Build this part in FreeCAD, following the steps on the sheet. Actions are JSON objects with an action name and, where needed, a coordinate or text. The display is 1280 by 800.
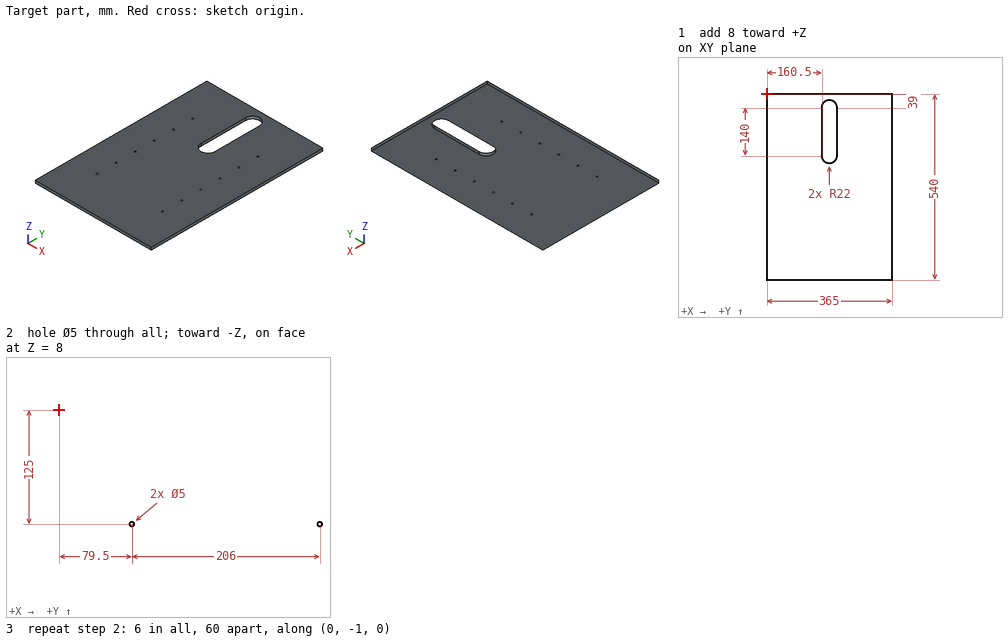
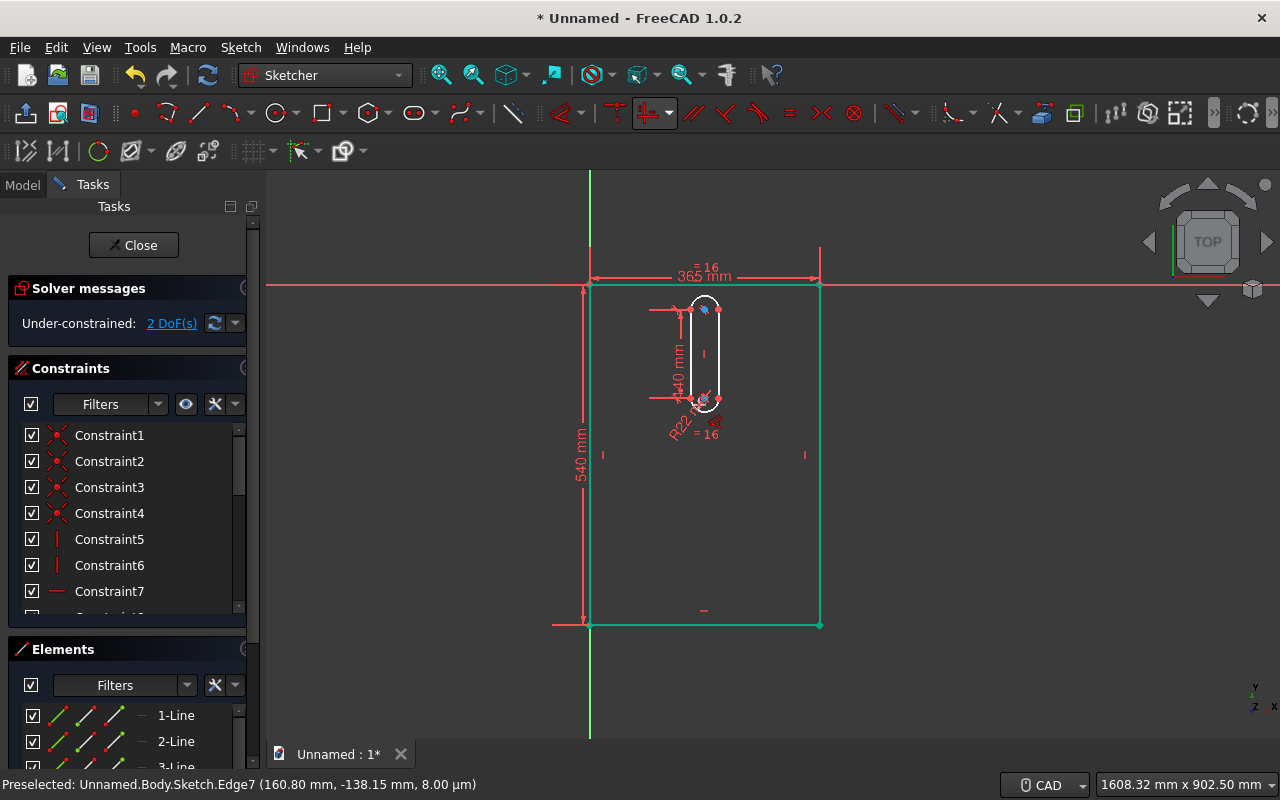
{"action": "scroll", "coordinate": [719, 310], "scroll_direction": "up", "scroll_amount": 3}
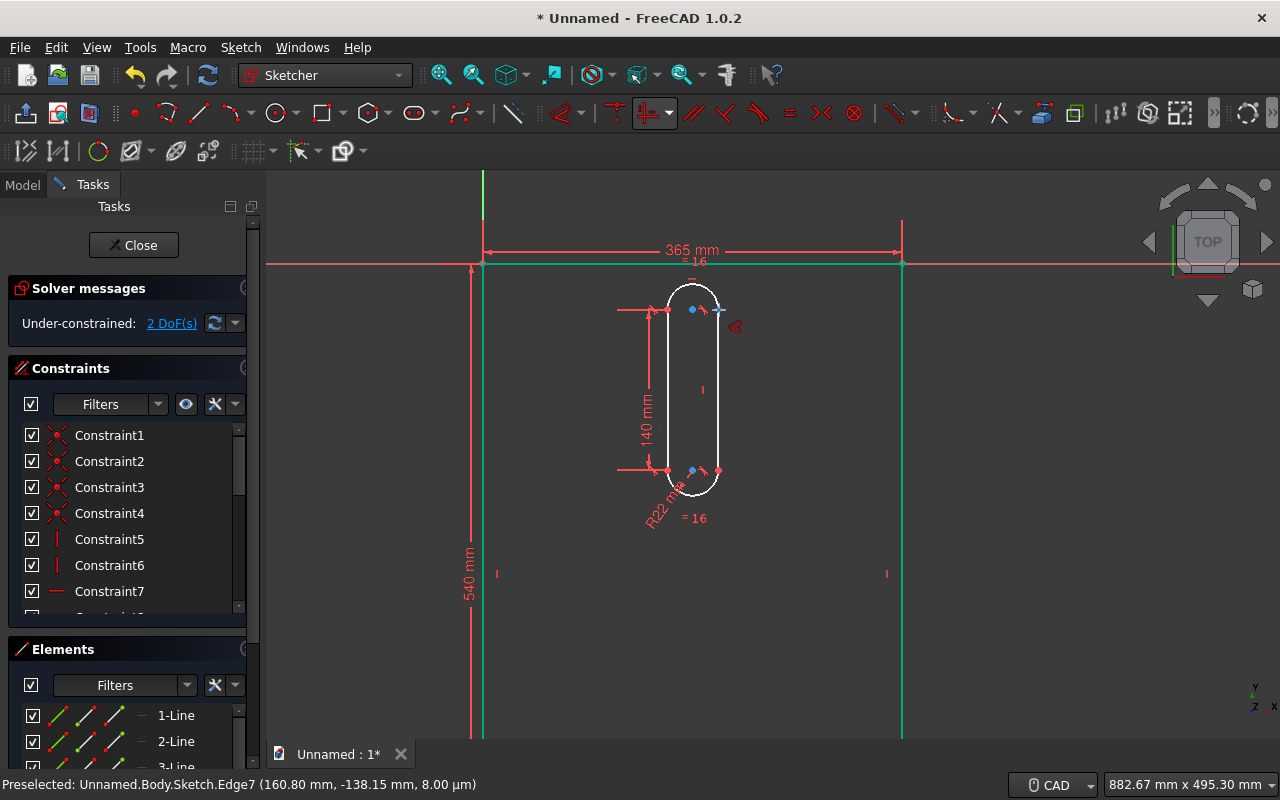
{"action": "left_click", "coordinate": [718, 310]}
{"action": "left_click", "coordinate": [449, 287]}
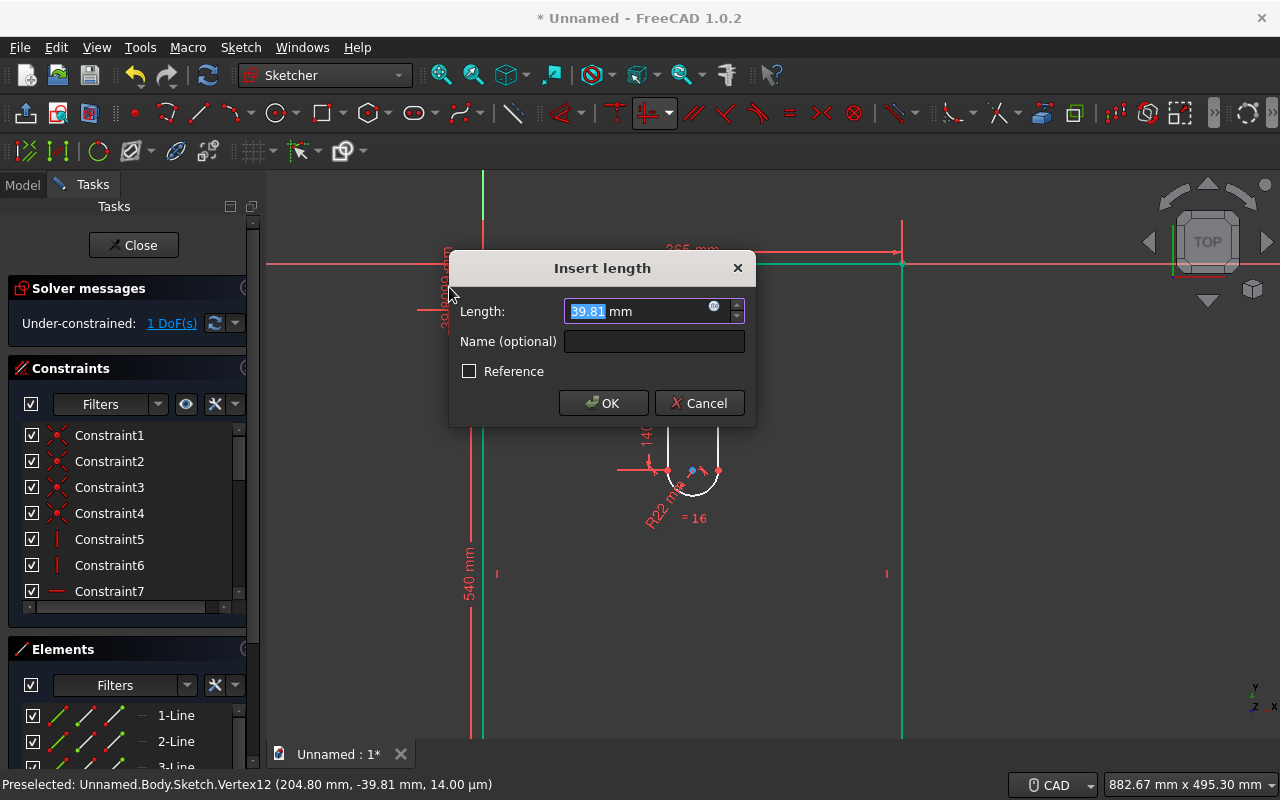
{"action": "type", "text": "39"}
{"action": "key", "text": "Return"}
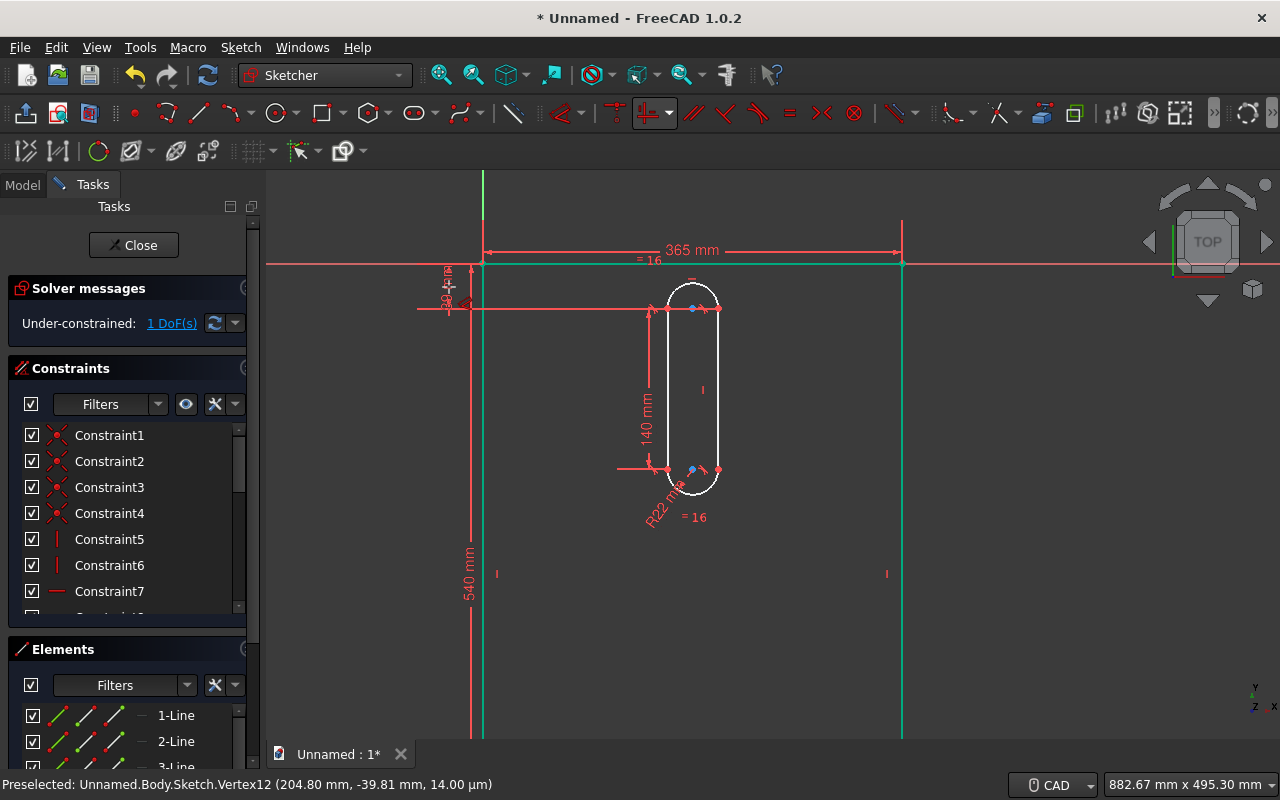
{"action": "left_click", "coordinate": [668, 469]}
{"action": "left_click", "coordinate": [575, 230]}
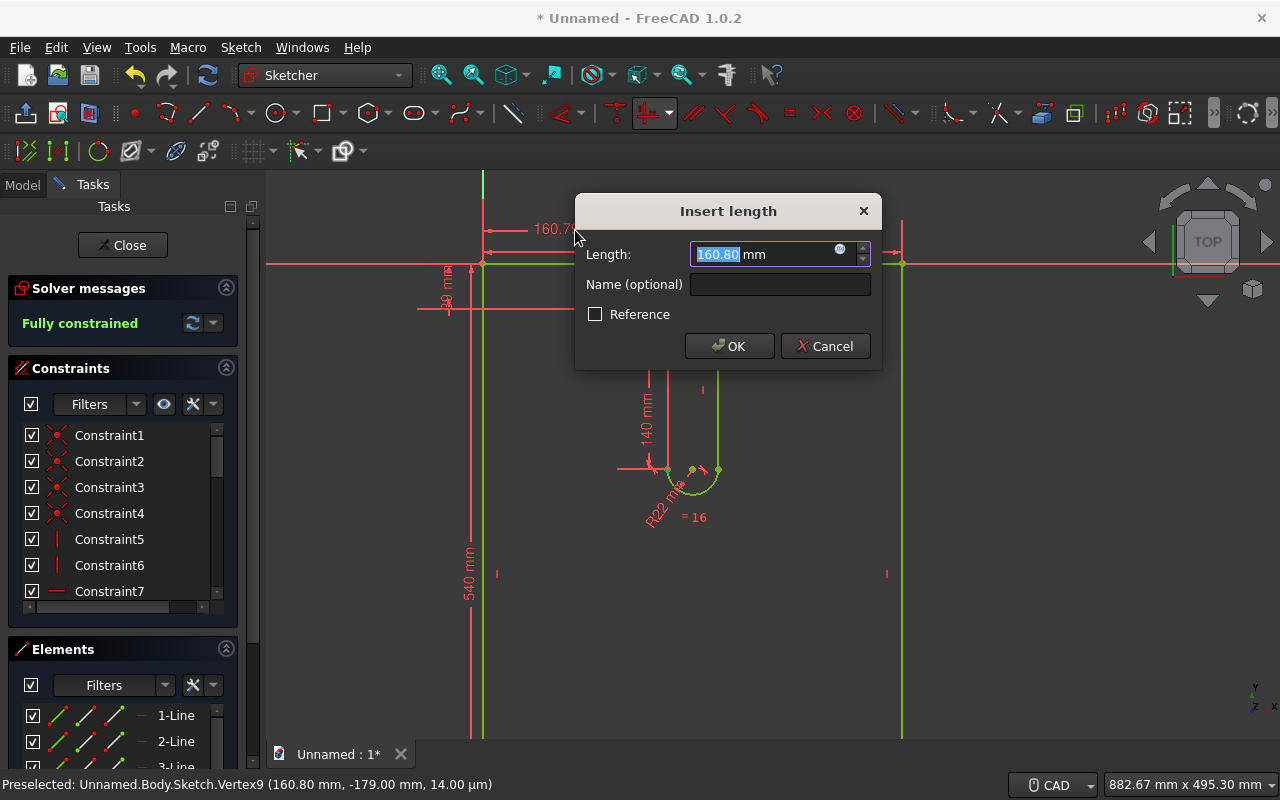
{"action": "type", "text": "160.5"}
{"action": "key", "text": "Return"}
{"action": "key", "text": "Escape"}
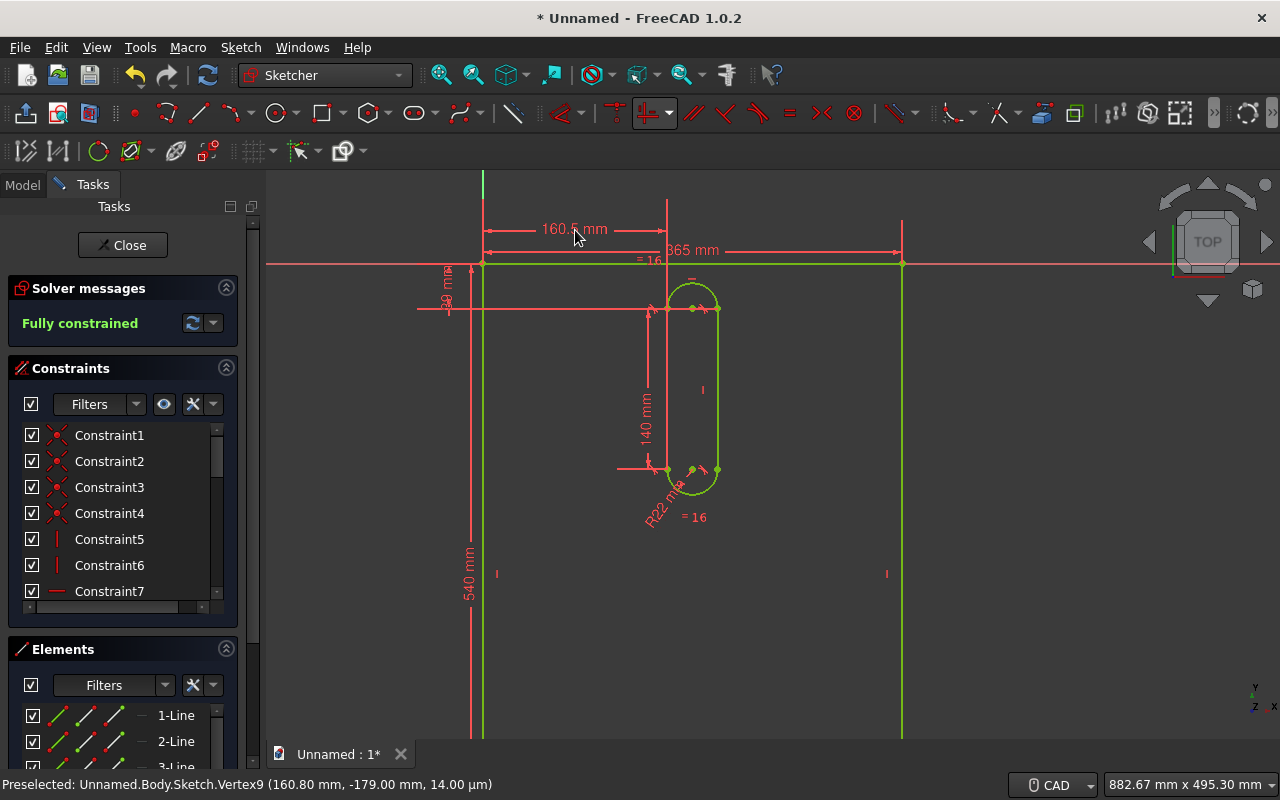
{"action": "left_click", "coordinate": [123, 245]}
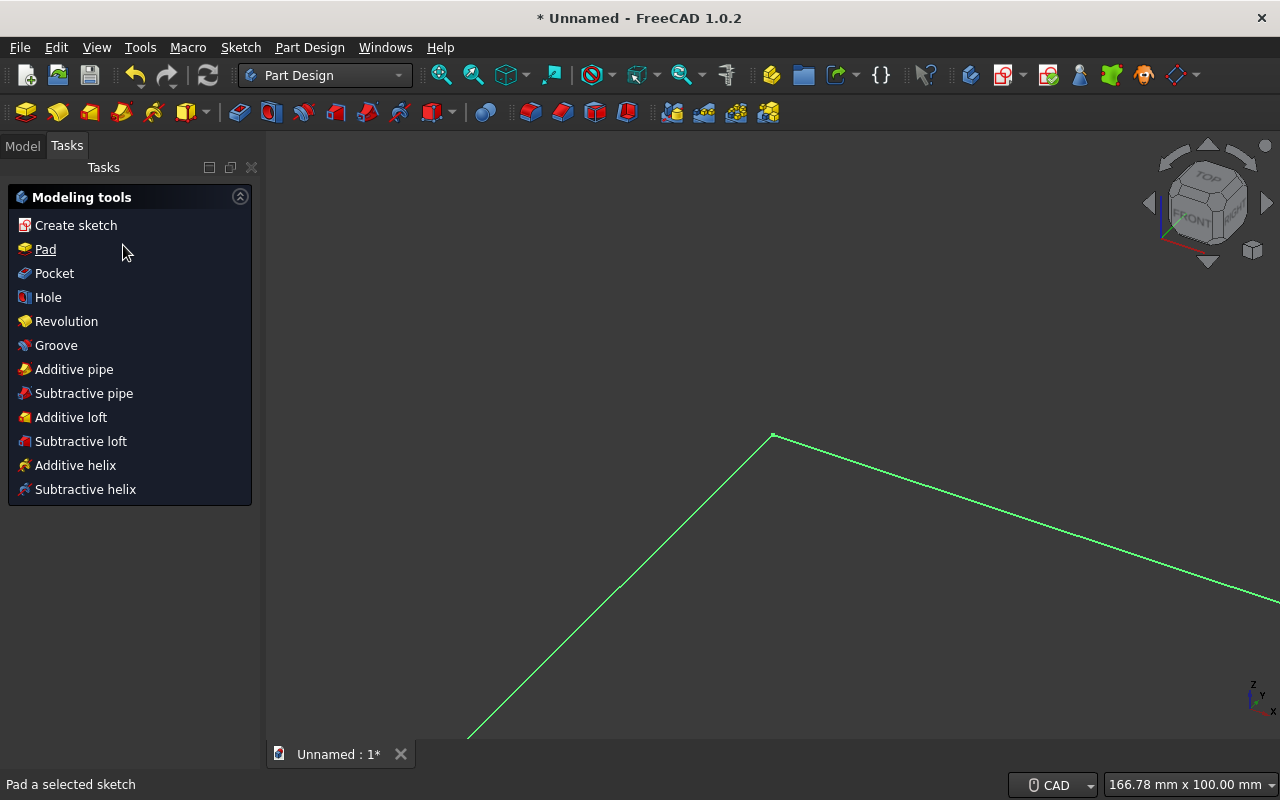
{"action": "left_click", "coordinate": [26, 112]}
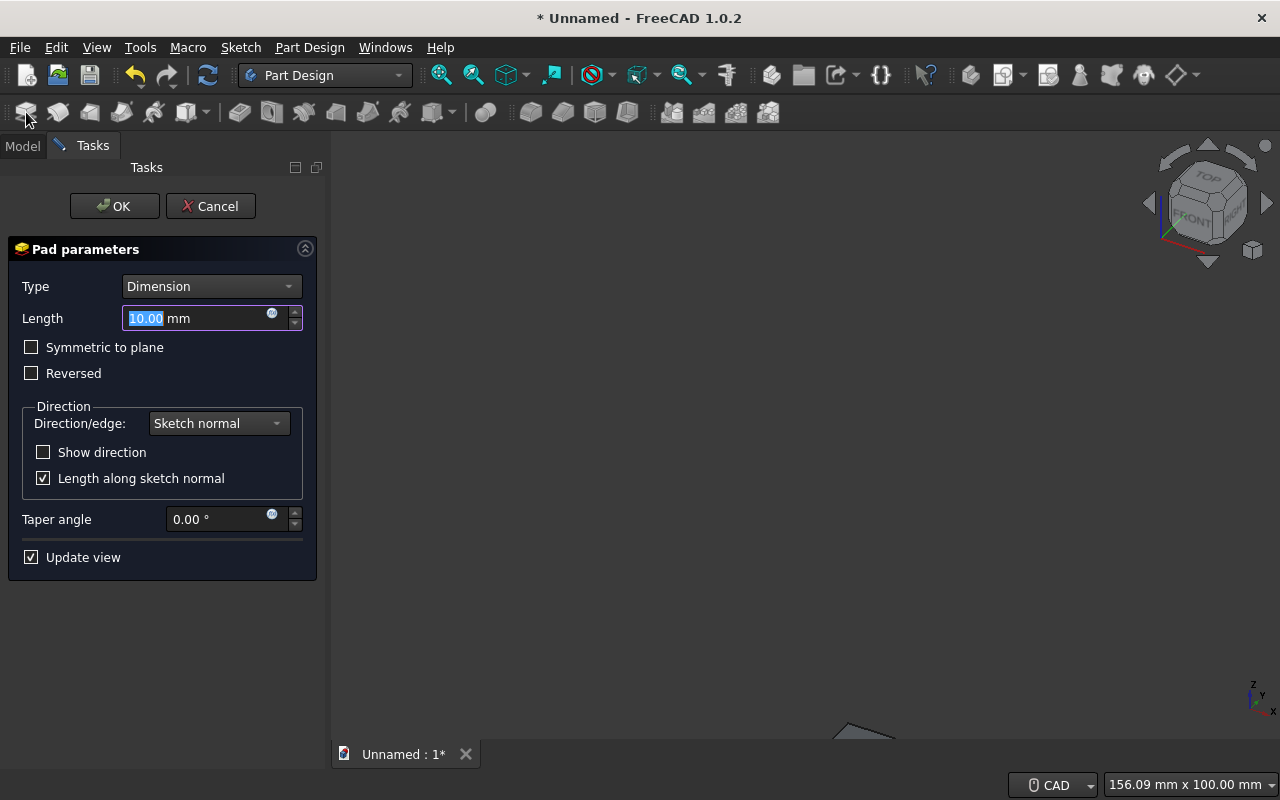
{"action": "type", "text": "8"}
{"action": "key", "text": "Tab"}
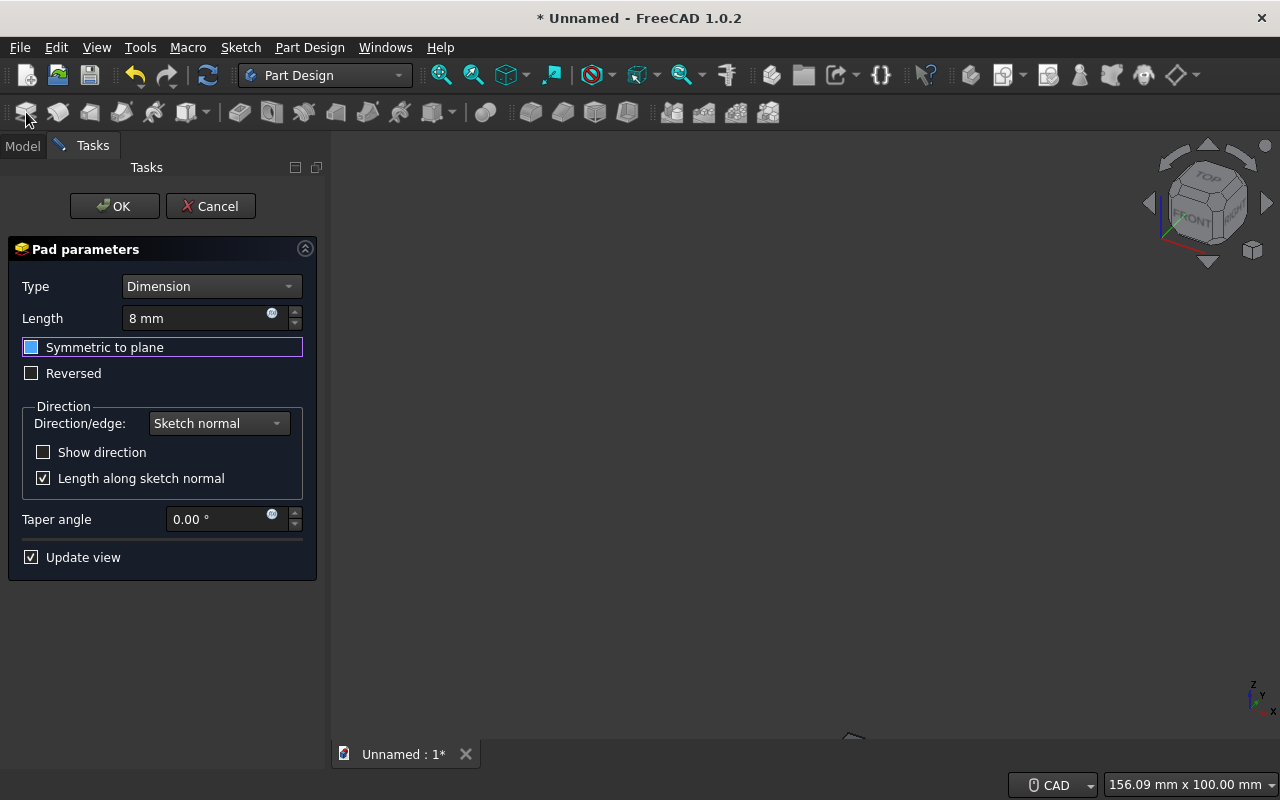
{"action": "left_click", "coordinate": [115, 206]}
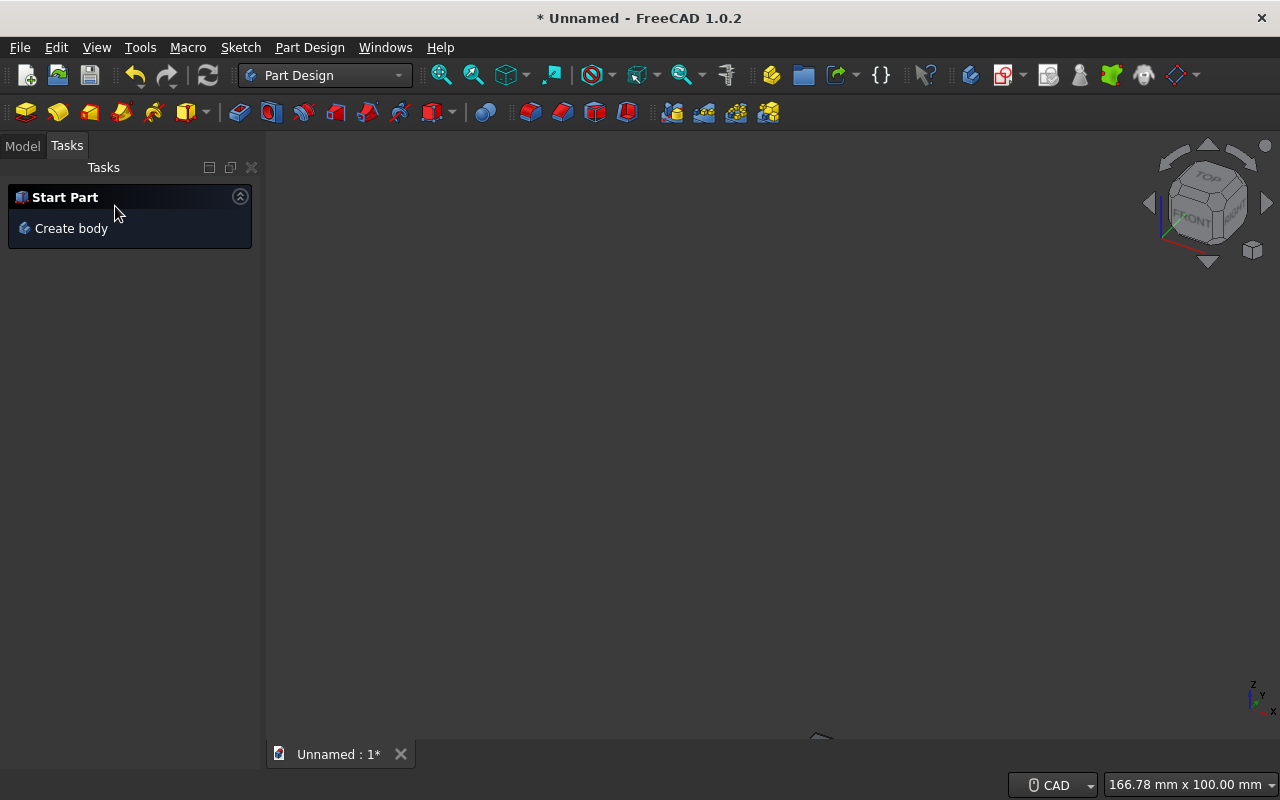
{"action": "left_click", "coordinate": [442, 76]}